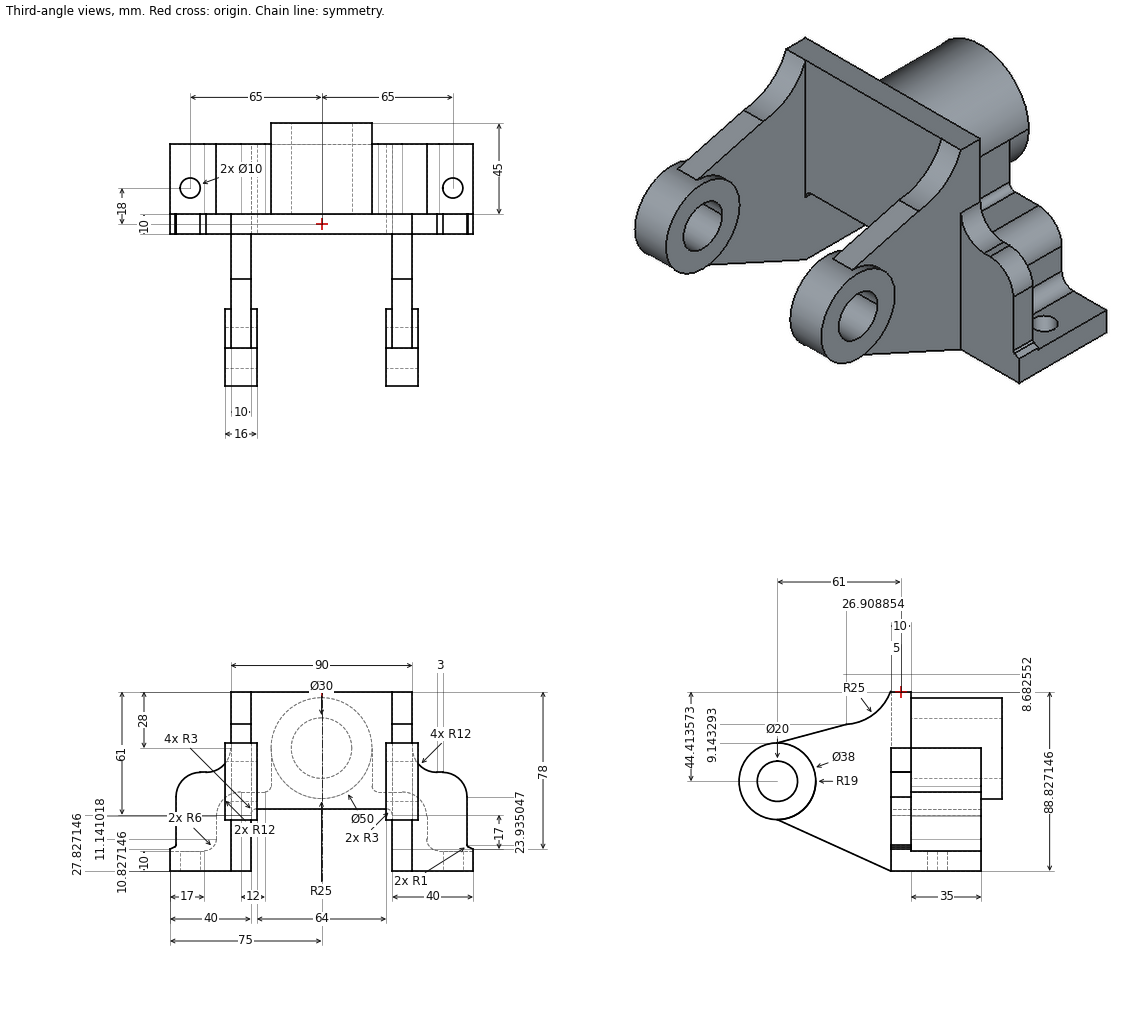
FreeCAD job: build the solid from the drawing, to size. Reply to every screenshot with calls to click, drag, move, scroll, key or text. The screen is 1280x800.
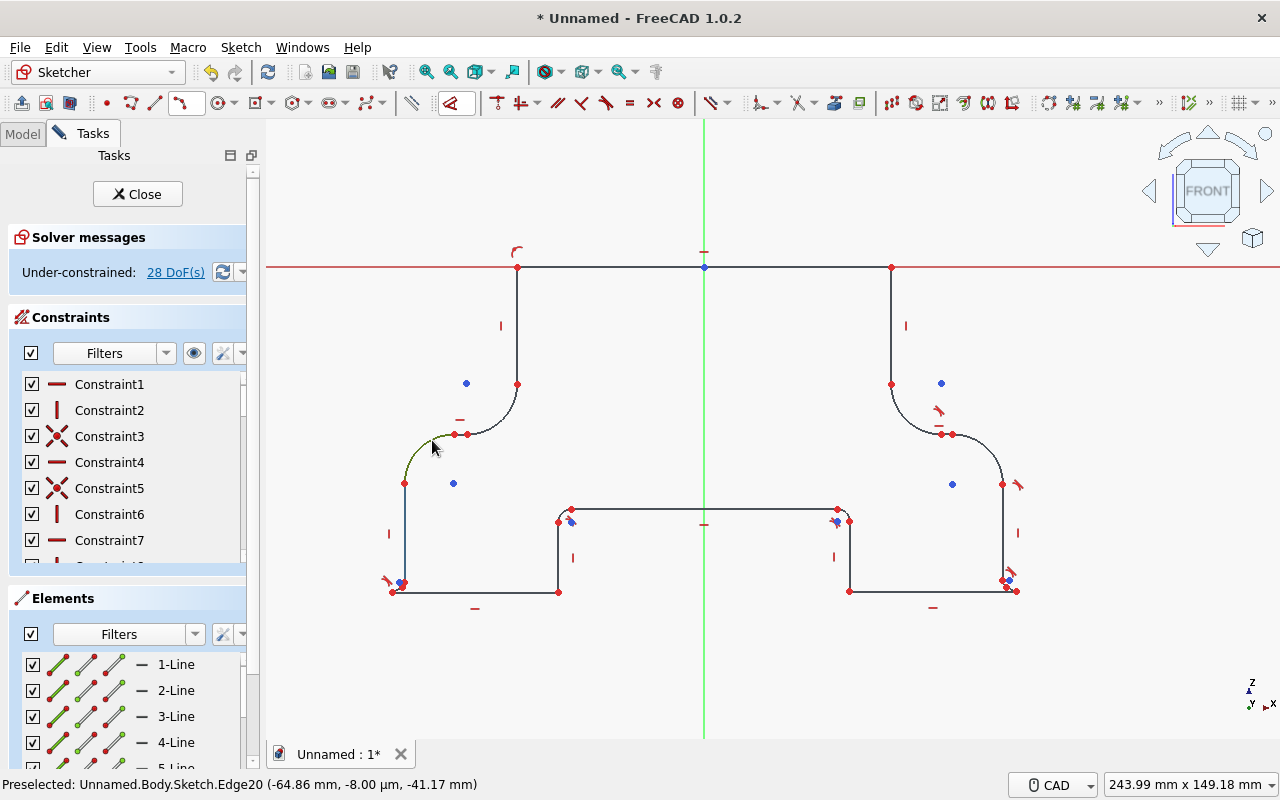
key(t)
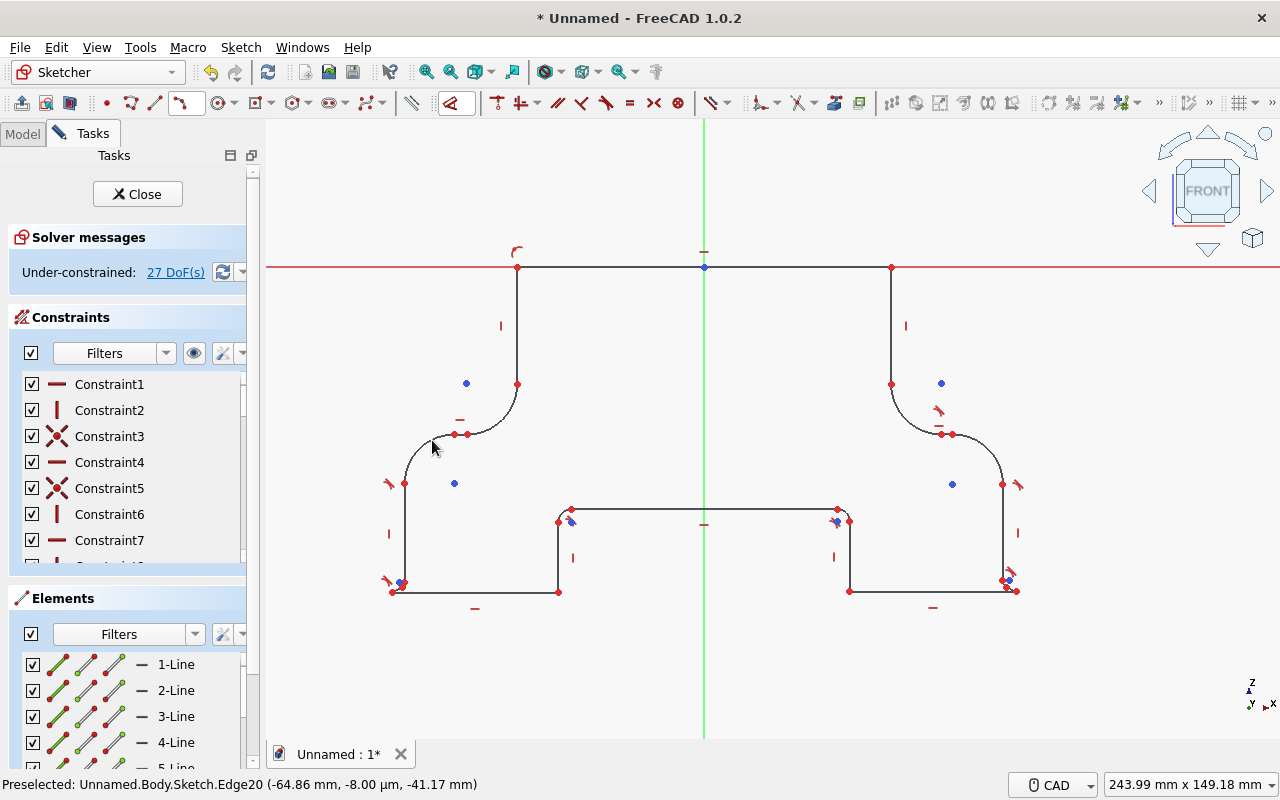
scroll(461, 435, up, 4)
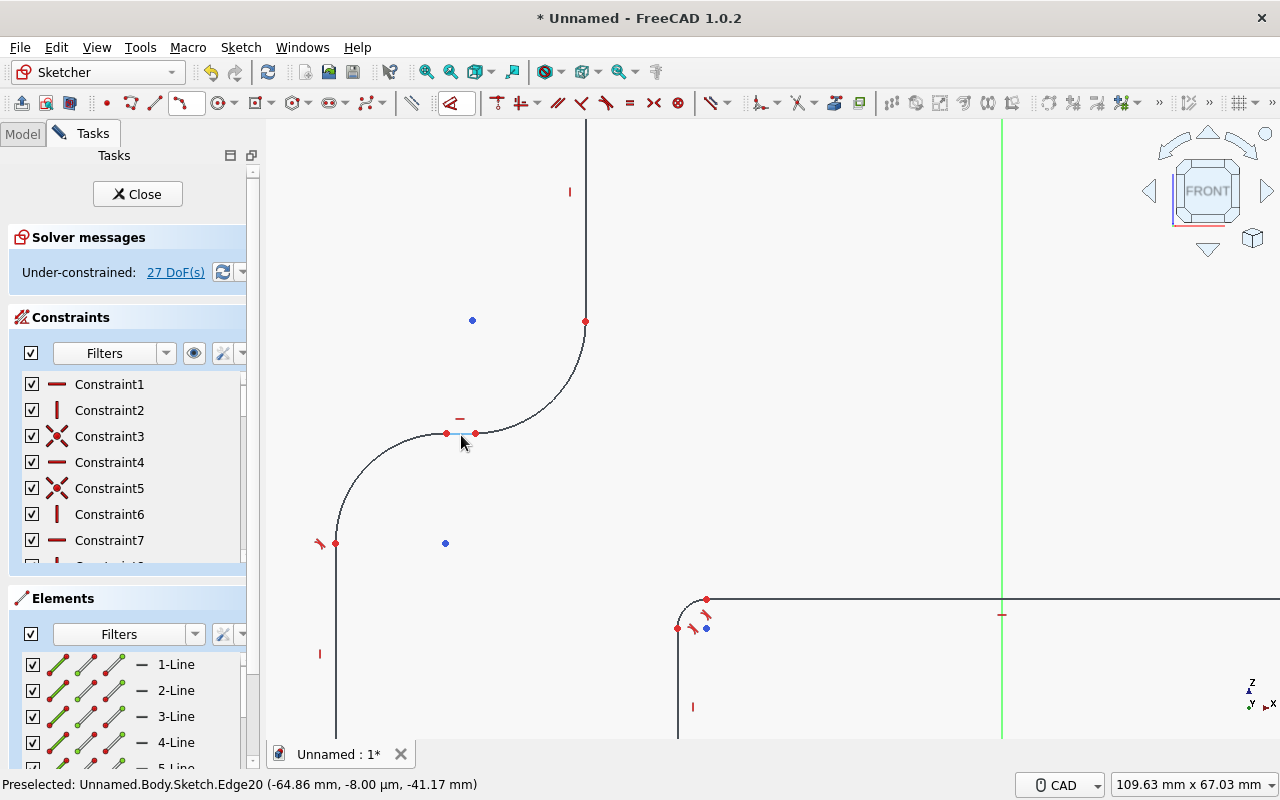
click(461, 434)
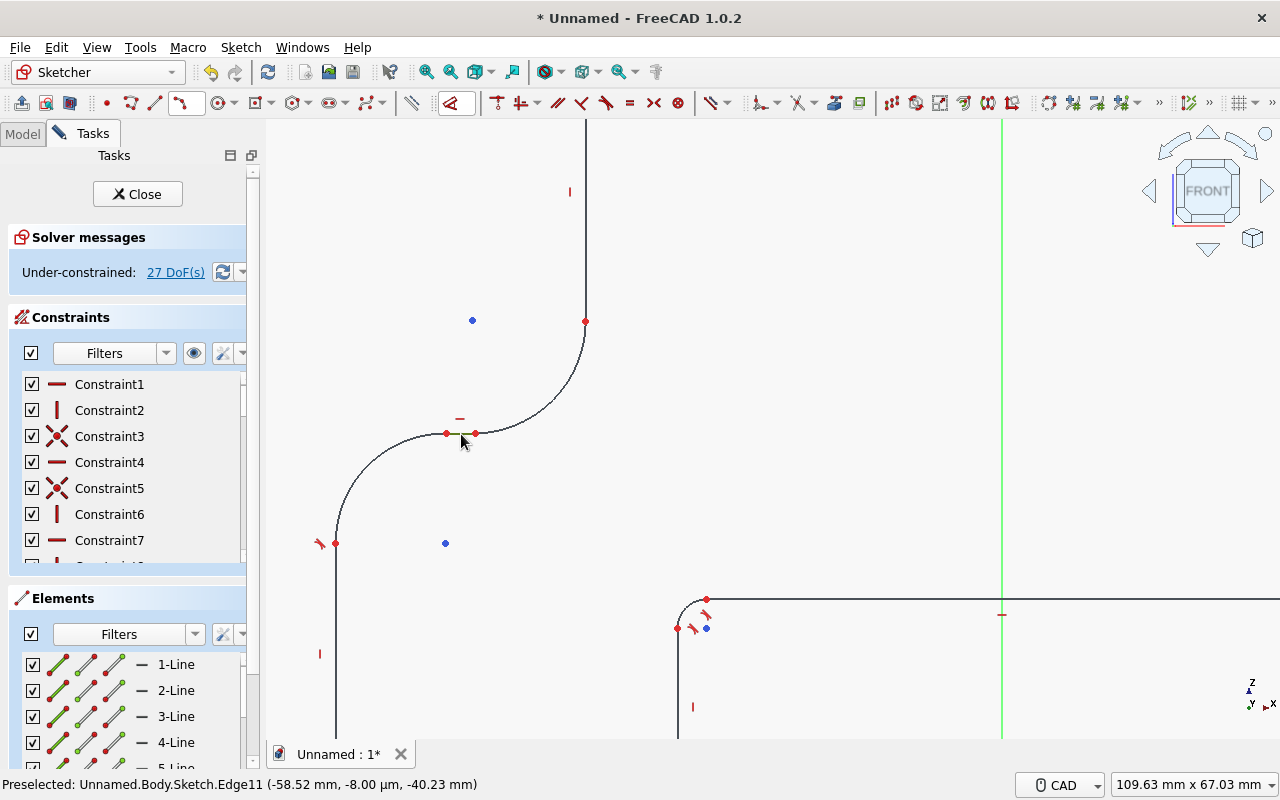
click(396, 445)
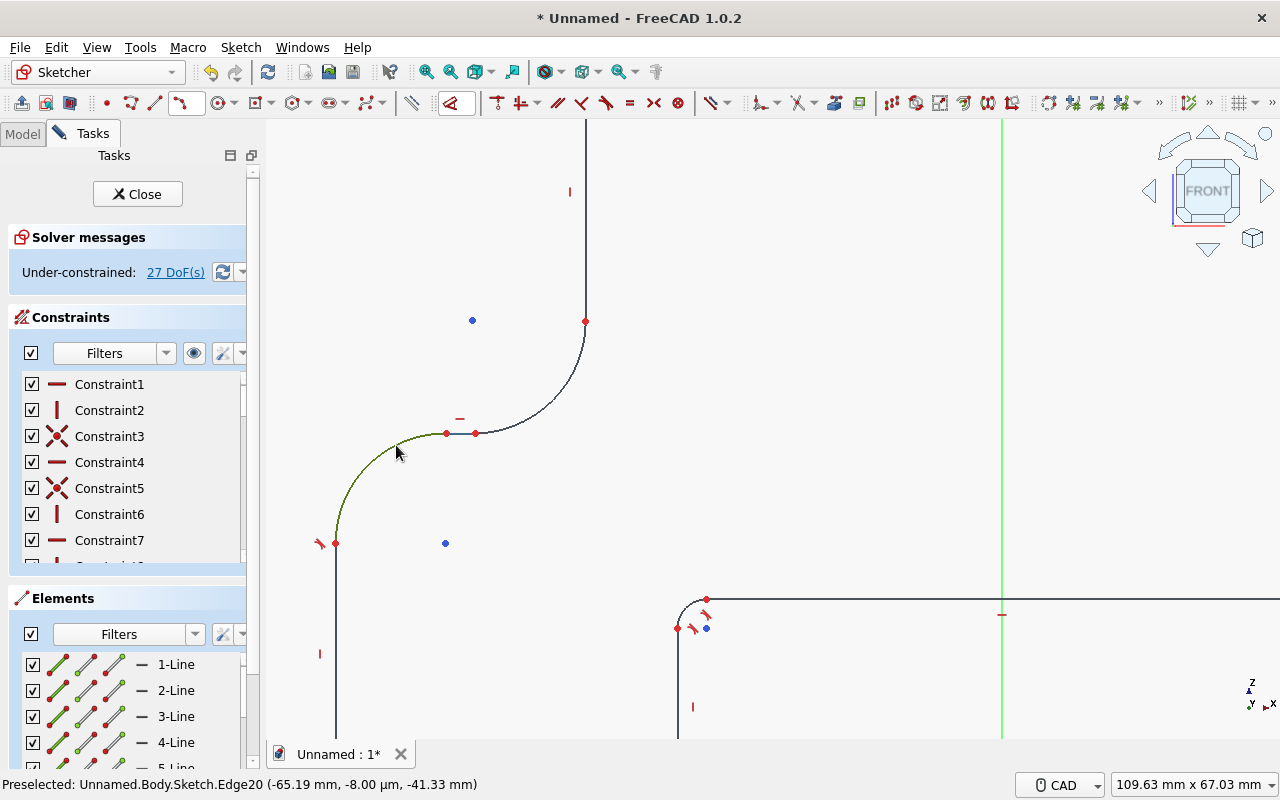
key(t)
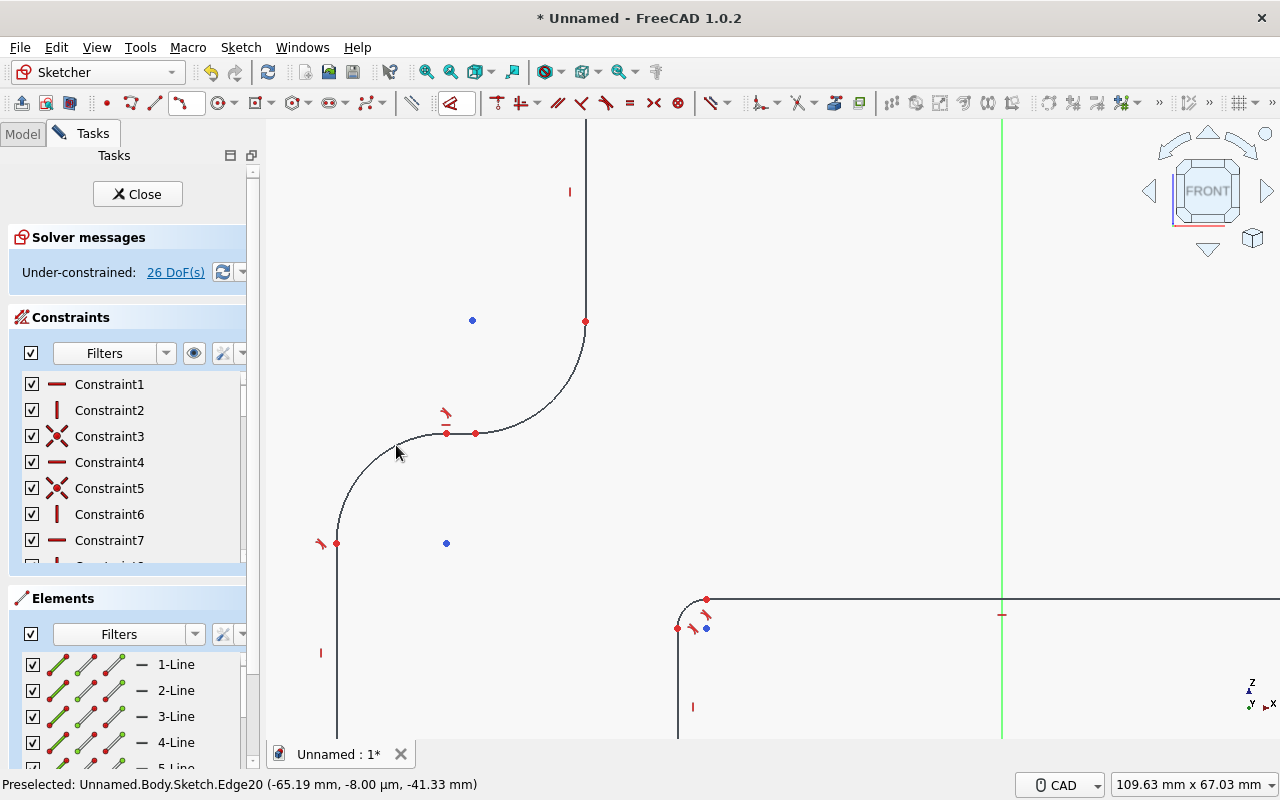
click(458, 434)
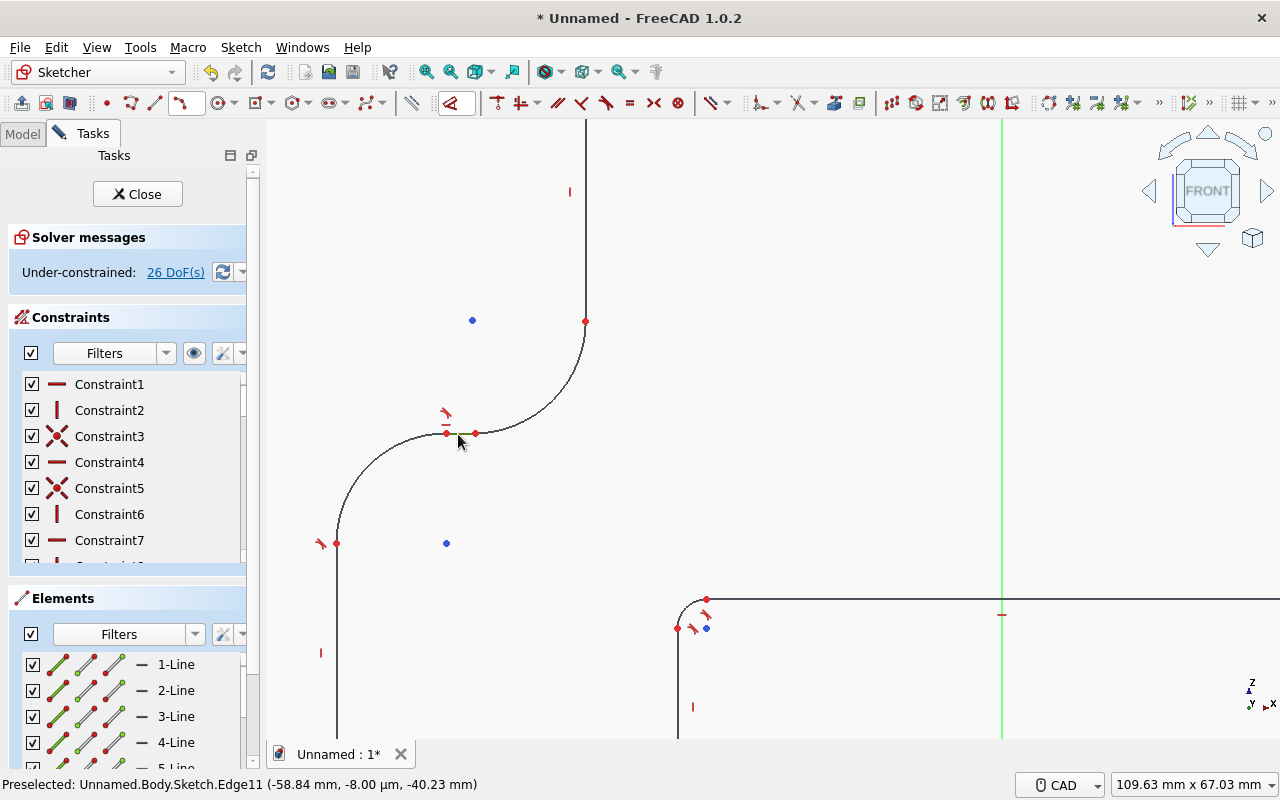
click(525, 421)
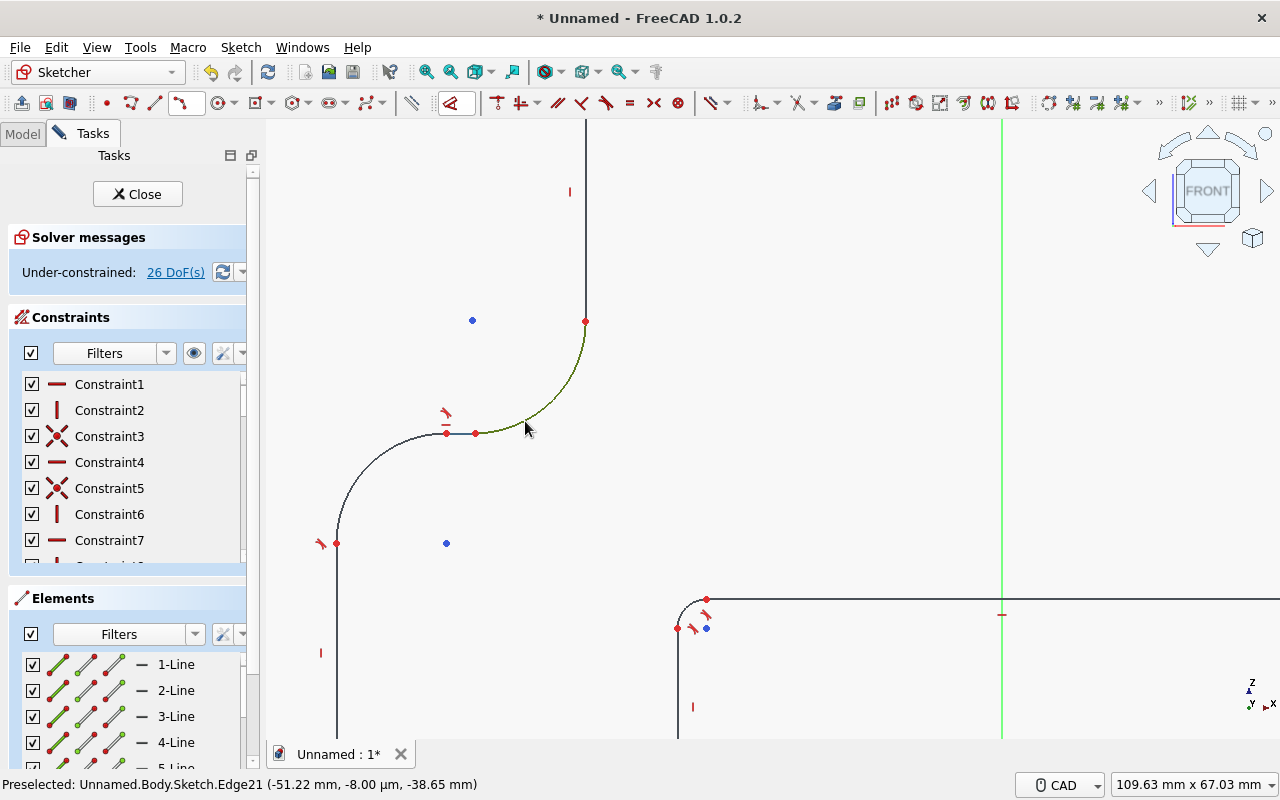
click(606, 104)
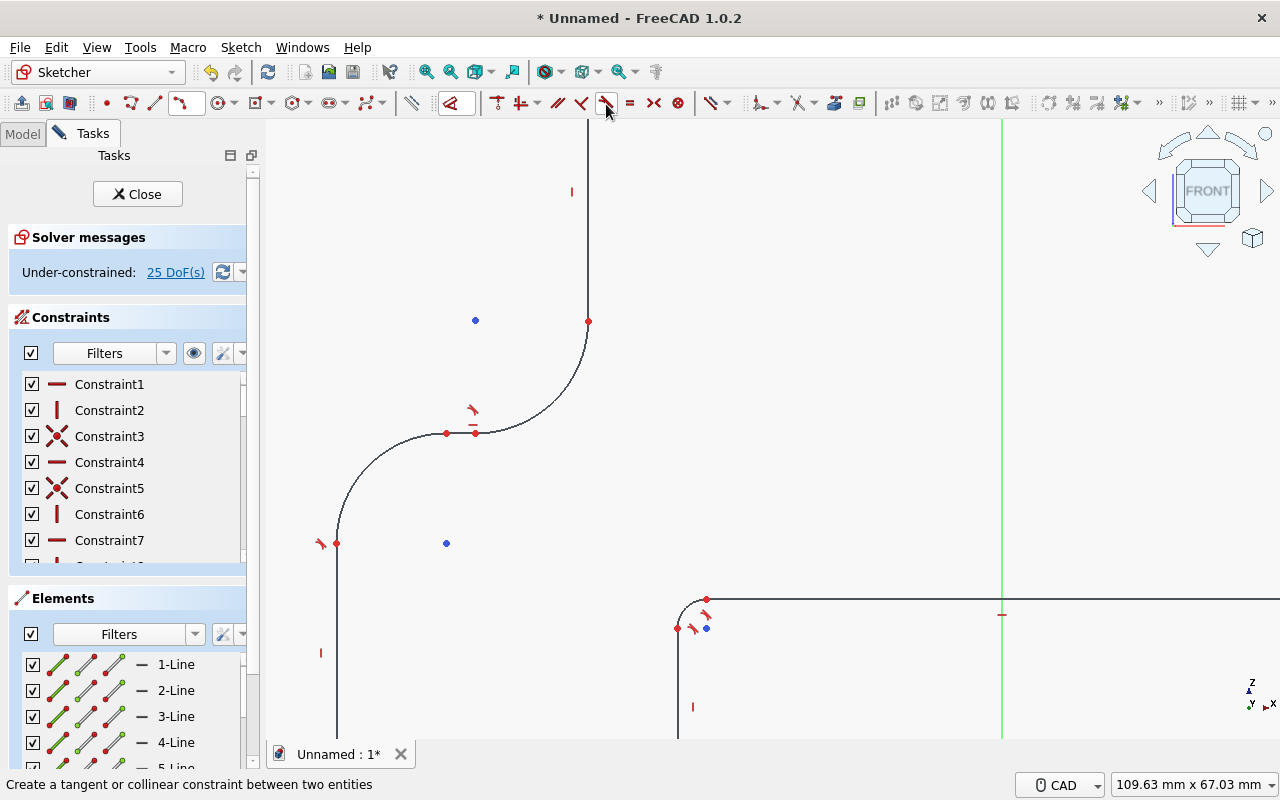
click(588, 243)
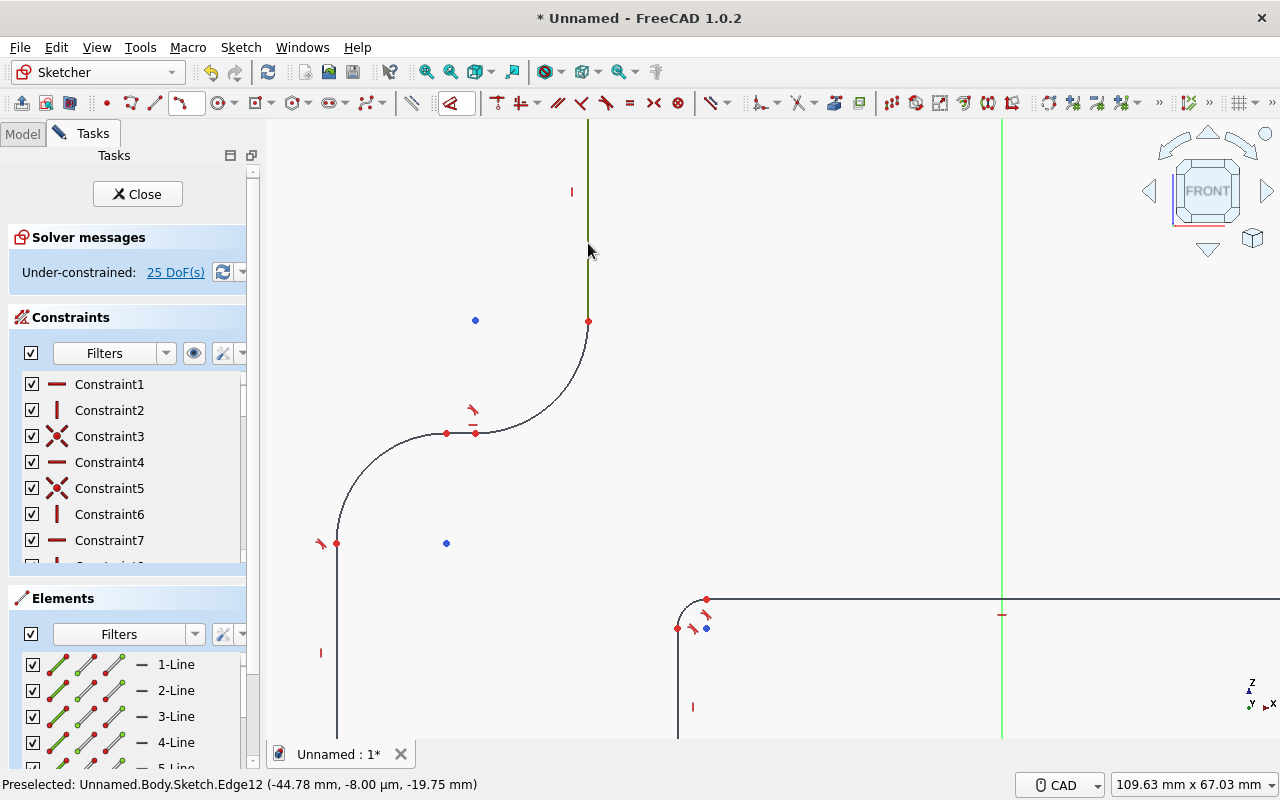
click(526, 421)